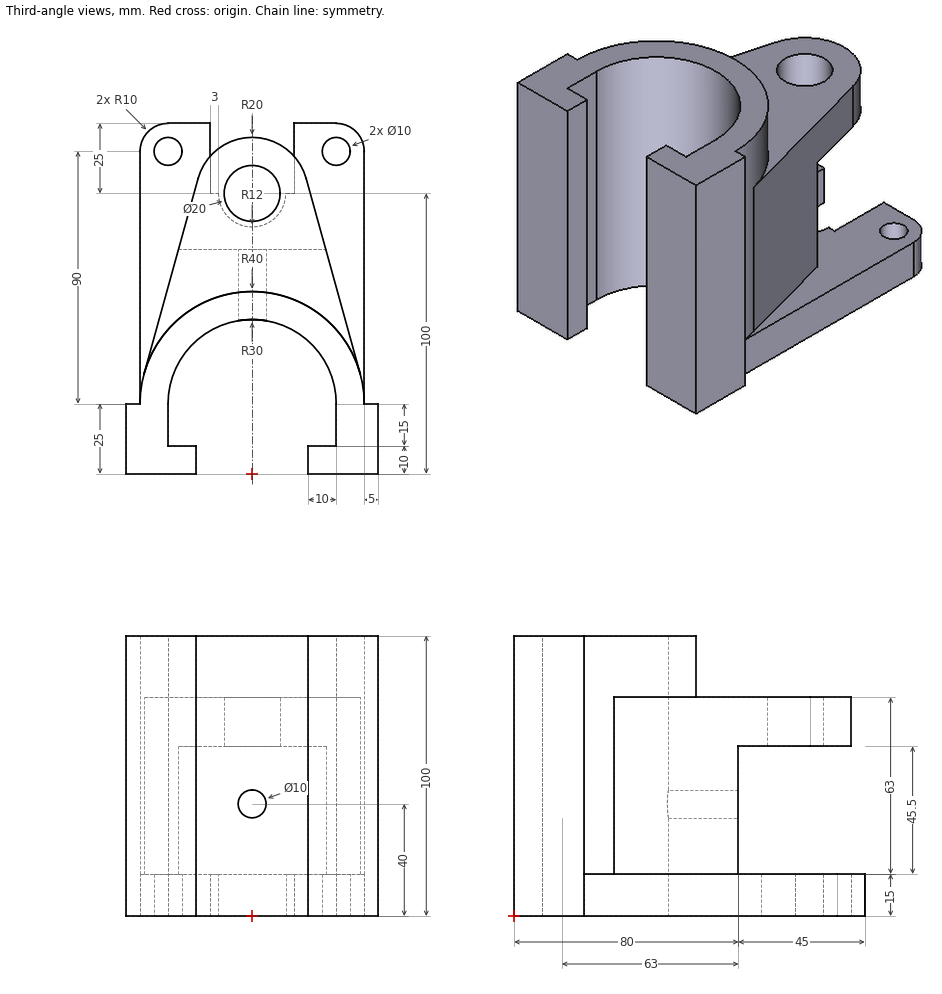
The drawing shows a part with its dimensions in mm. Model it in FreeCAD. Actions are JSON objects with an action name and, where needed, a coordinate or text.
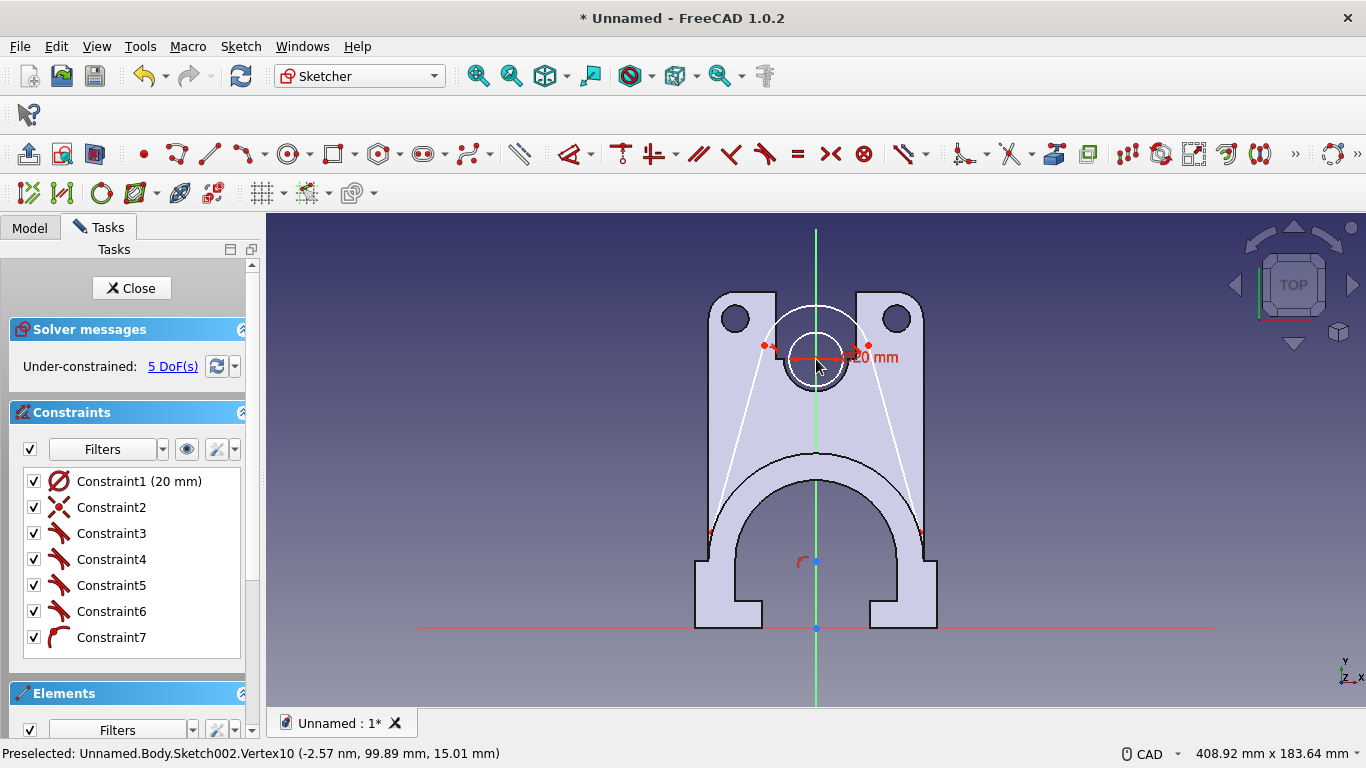
{"action": "left_click", "coordinate": [816, 585]}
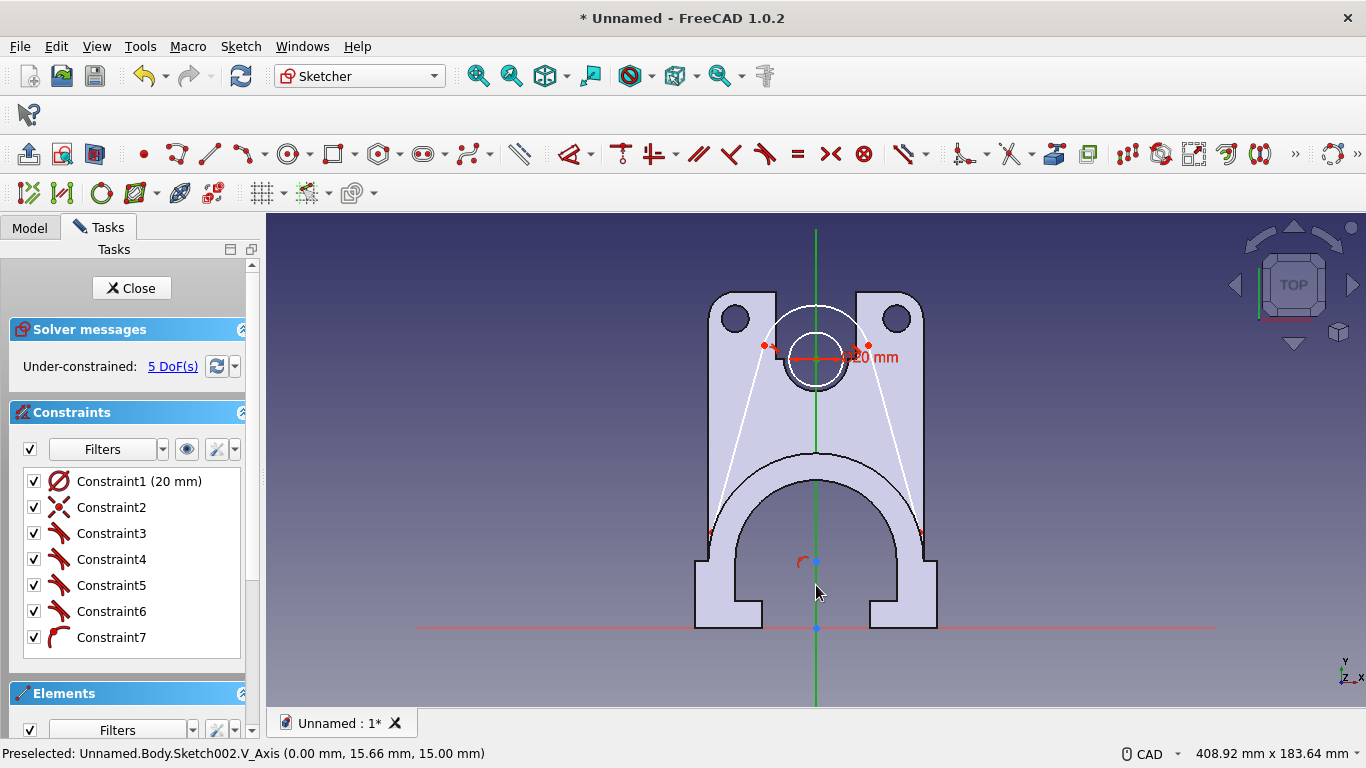
{"action": "key", "text": "c"}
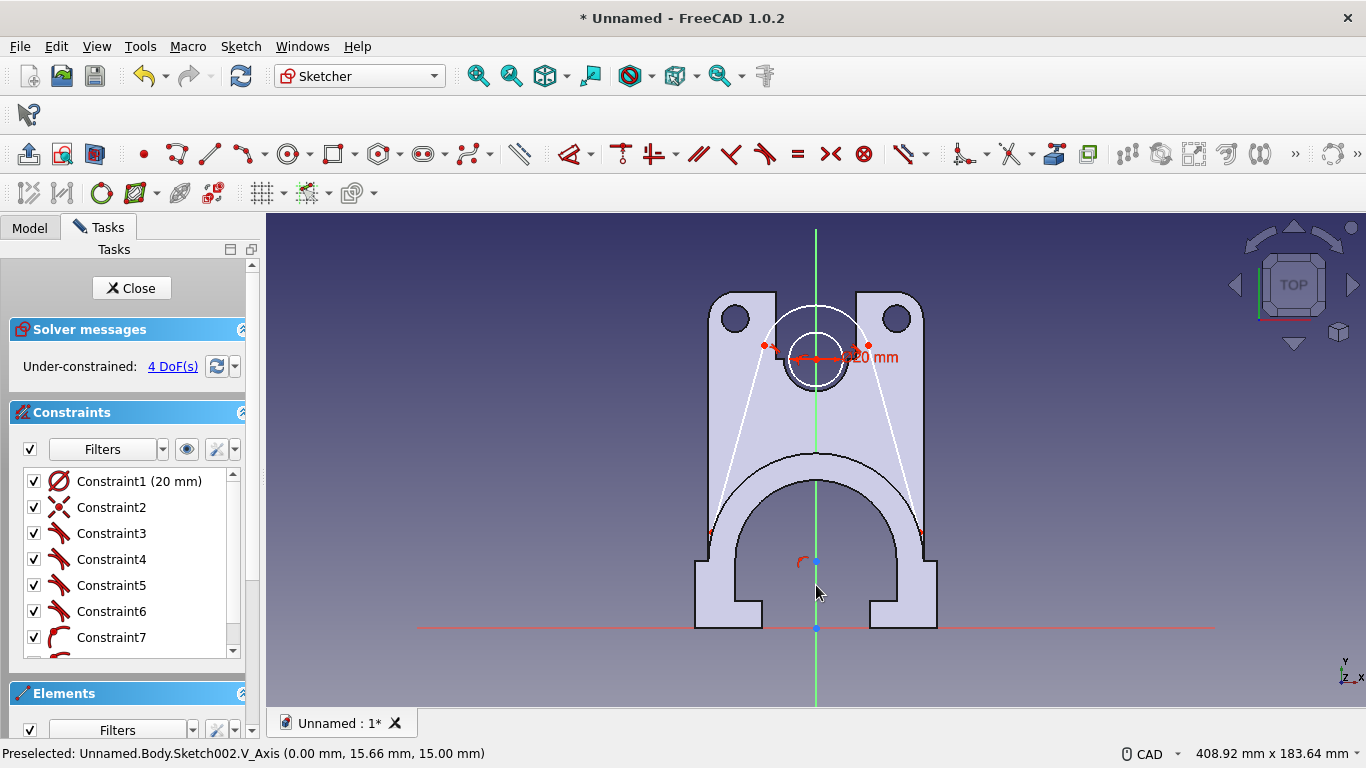
{"action": "left_click", "coordinate": [568, 154]}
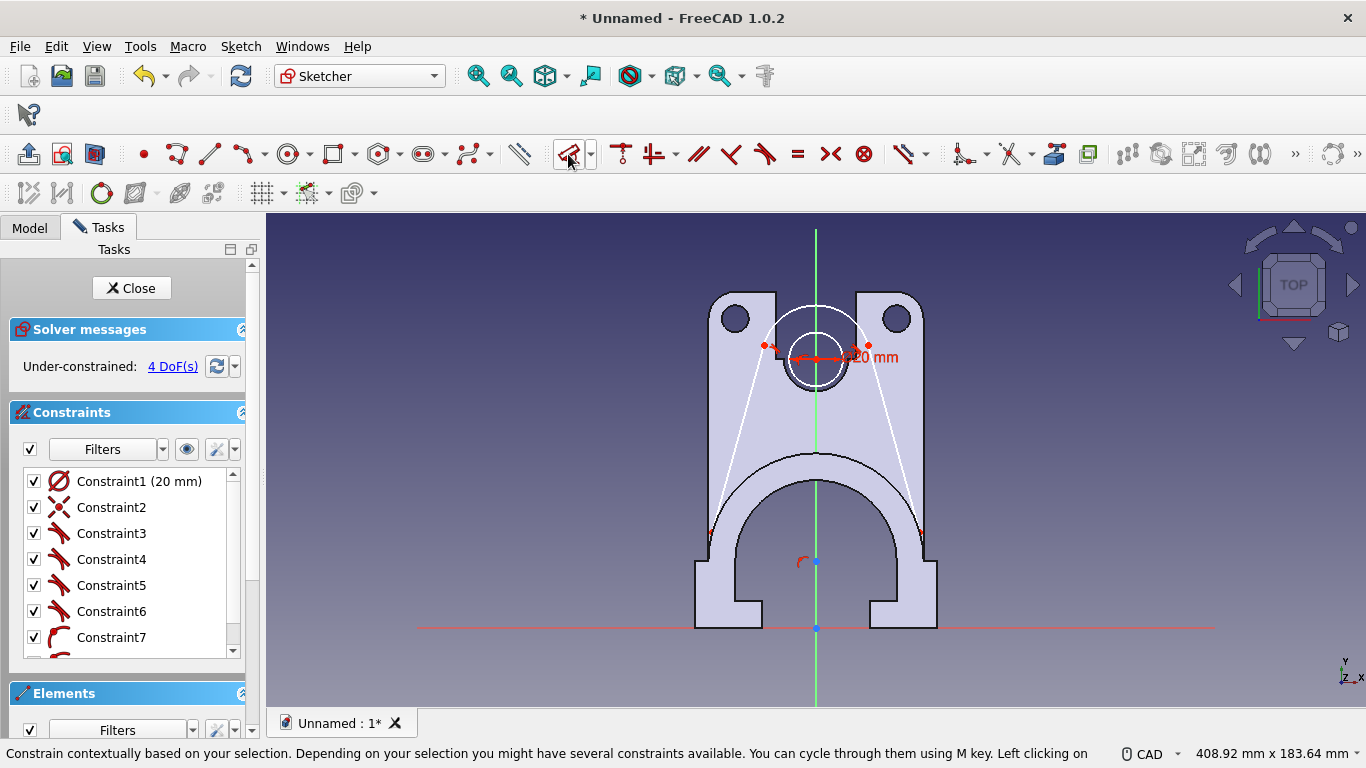
{"action": "left_click", "coordinate": [870, 468]}
{"action": "left_click", "coordinate": [936, 489]}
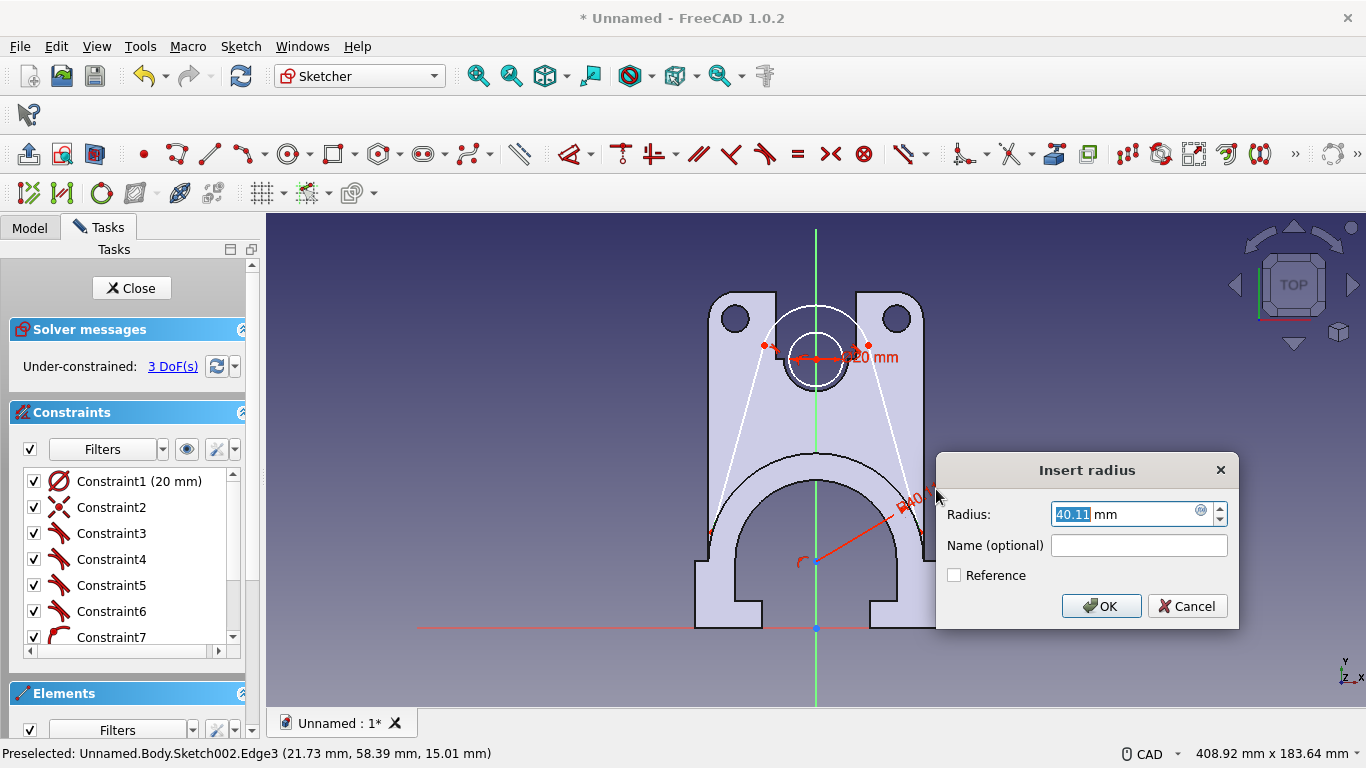
{"action": "type", "text": "40"}
{"action": "key", "text": "Return"}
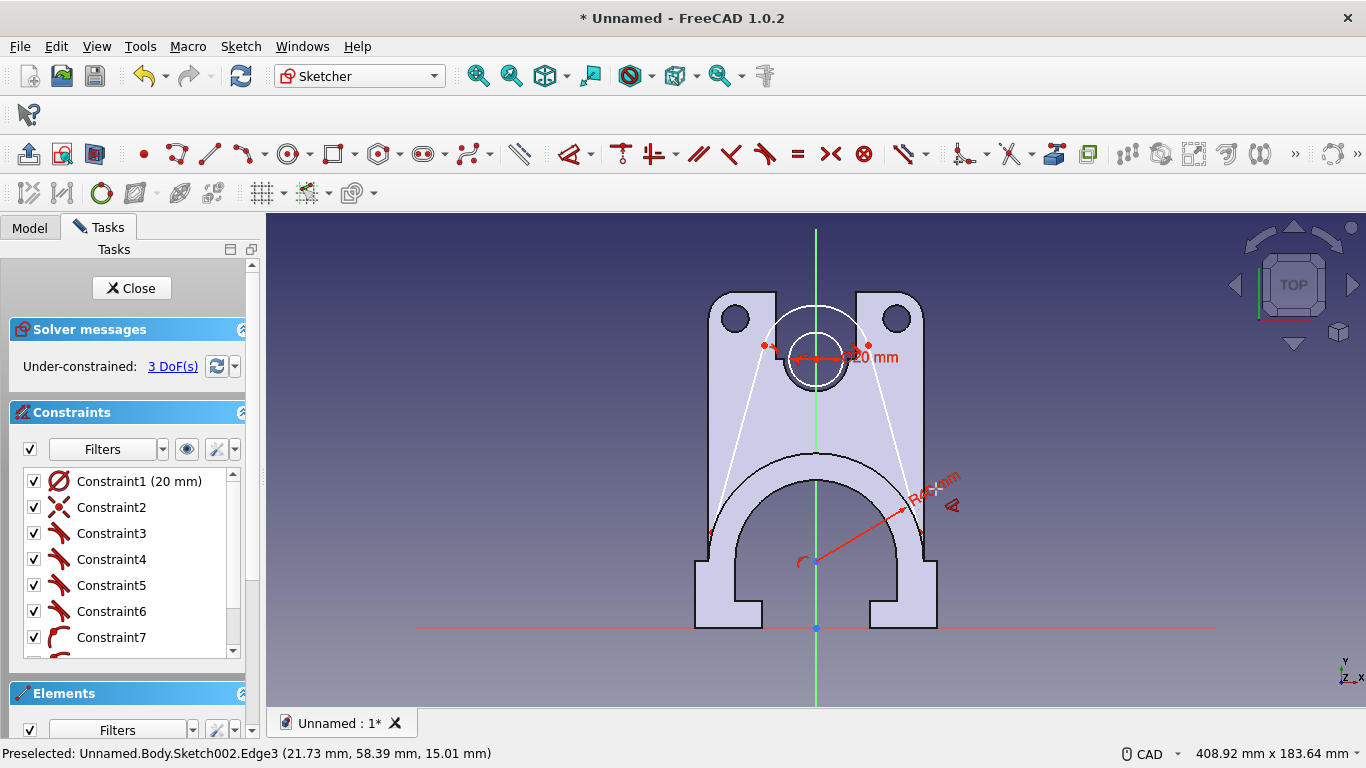
{"action": "left_click", "coordinate": [843, 313]}
{"action": "left_click", "coordinate": [859, 285]}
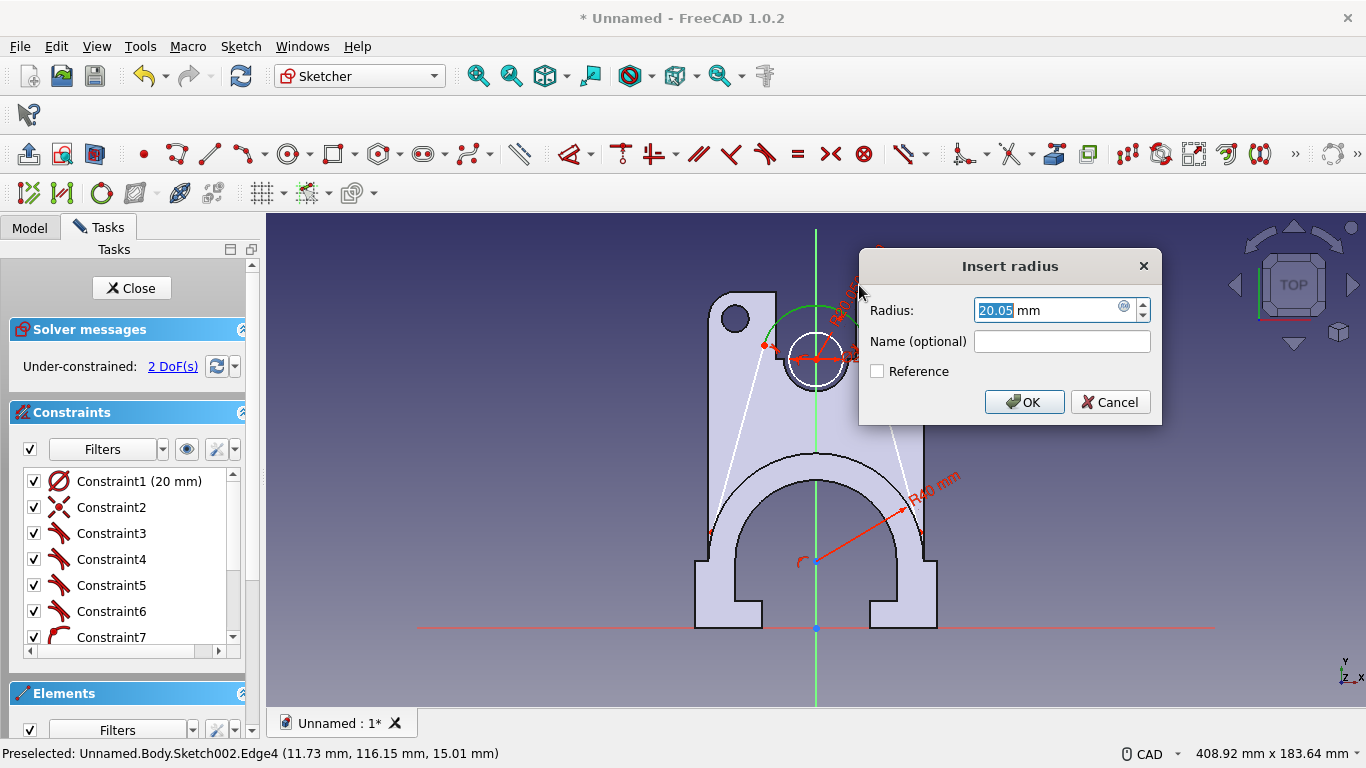
{"action": "type", "text": "20"}
{"action": "key", "text": "Return"}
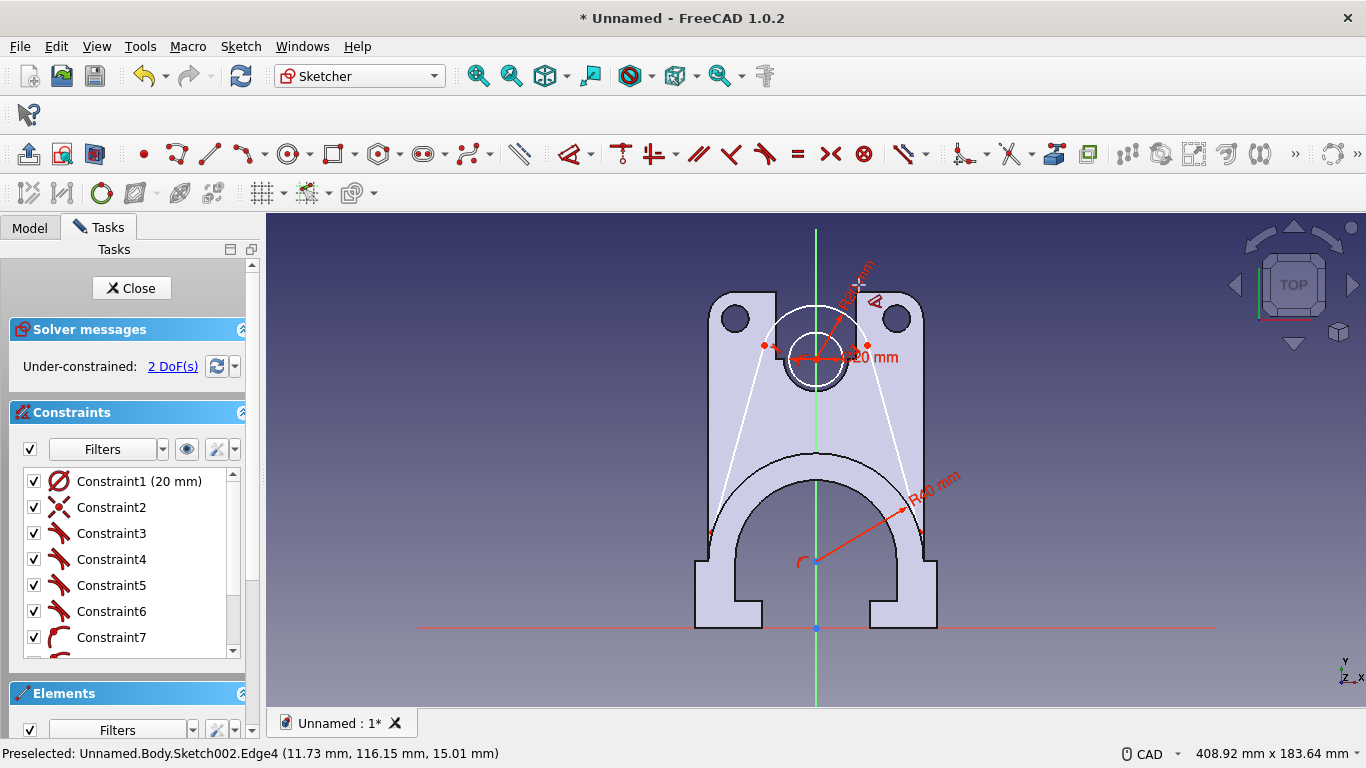
{"action": "left_click", "coordinate": [816, 562]}
{"action": "left_click", "coordinate": [850, 595]}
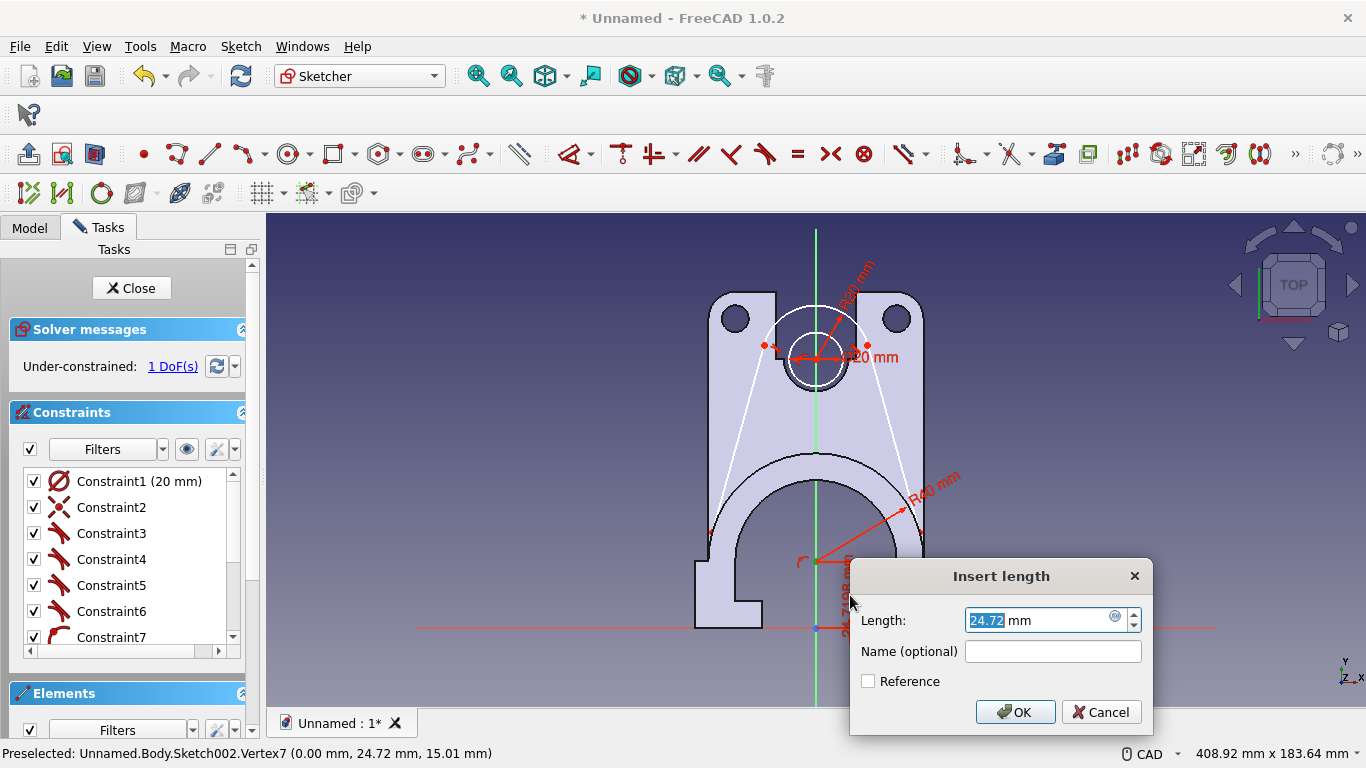
{"action": "type", "text": "25"}
{"action": "key", "text": "Return"}